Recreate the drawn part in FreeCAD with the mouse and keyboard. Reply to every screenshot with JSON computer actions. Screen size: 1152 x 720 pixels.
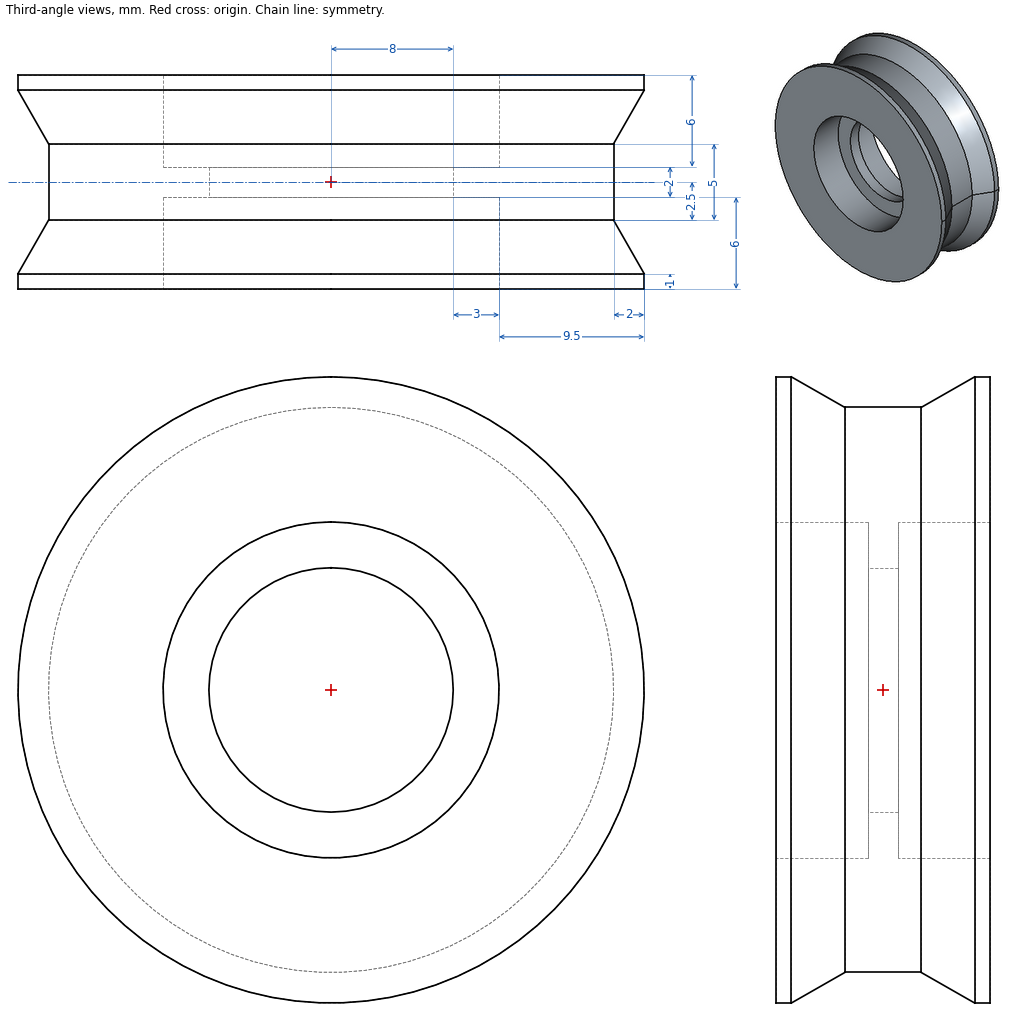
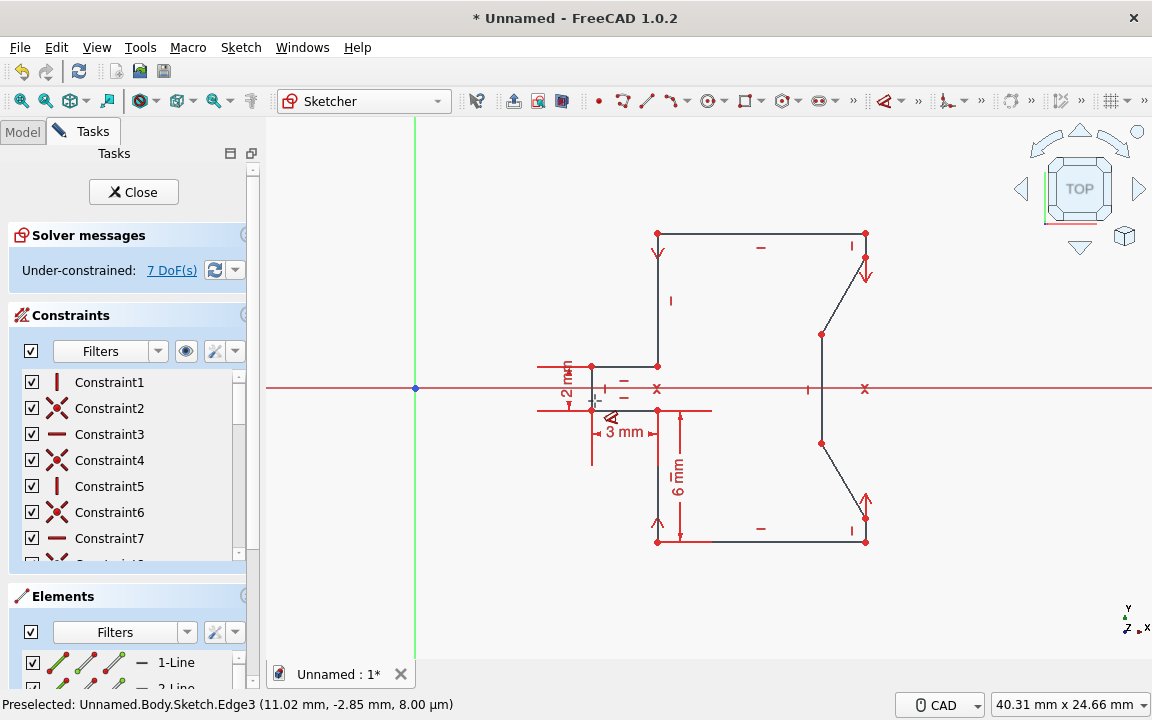
{"action": "scroll", "coordinate": [866, 535], "scroll_direction": "up", "scroll_amount": 4}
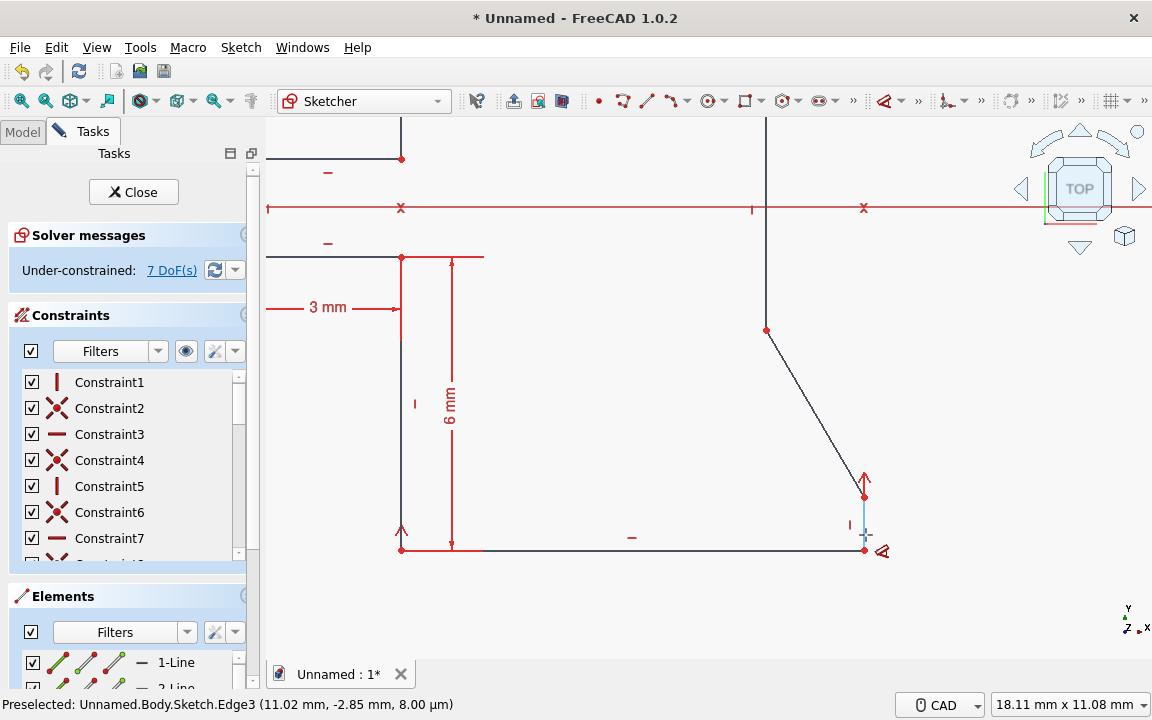
{"action": "left_click", "coordinate": [864, 535]}
{"action": "left_click", "coordinate": [898, 524]}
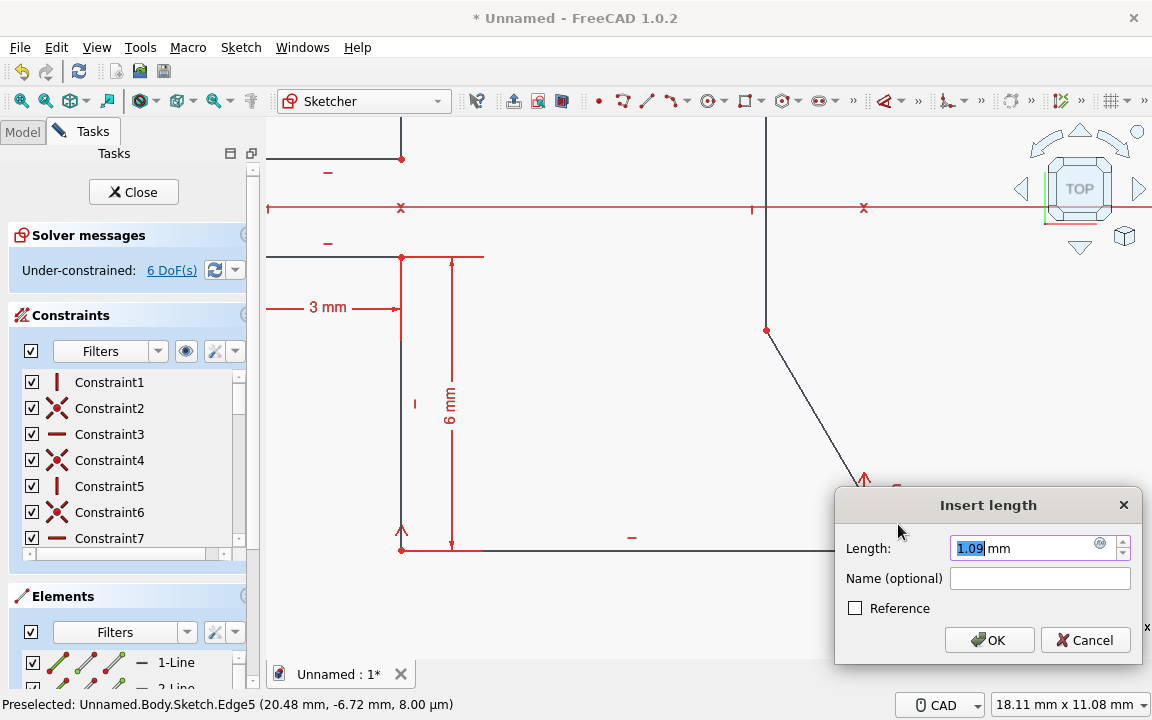
{"action": "type", "text": "1"}
{"action": "key", "text": "Return"}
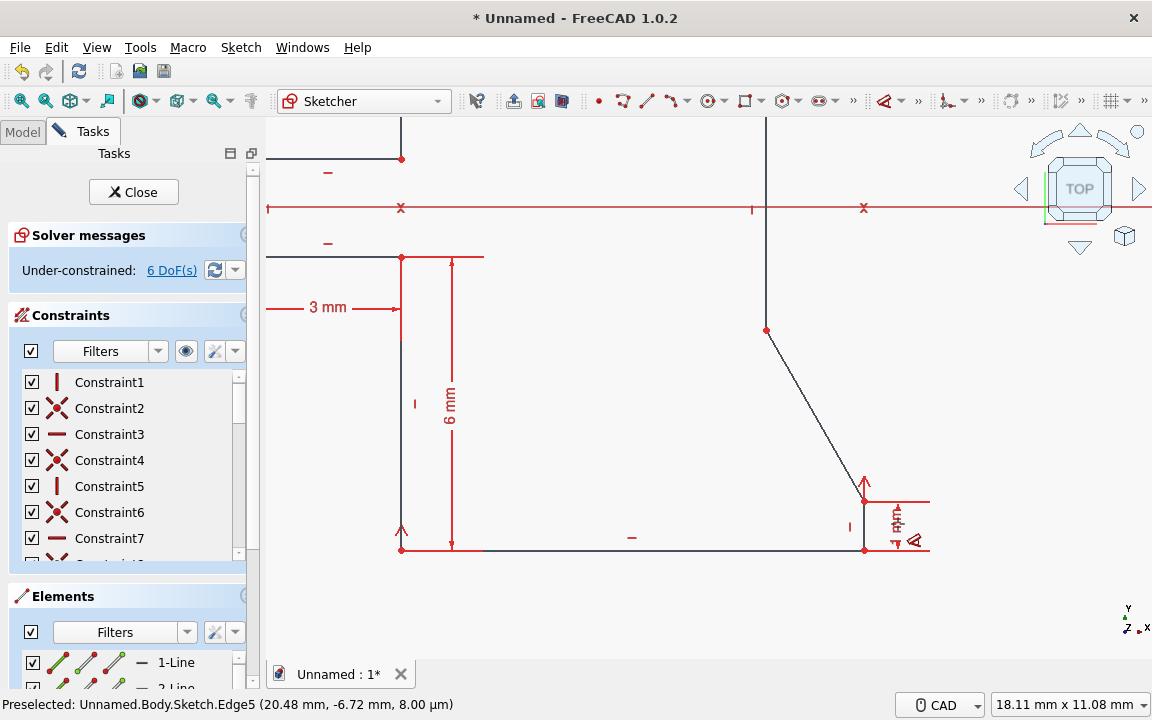
{"action": "left_click", "coordinate": [766, 258]}
{"action": "left_click", "coordinate": [800, 238]}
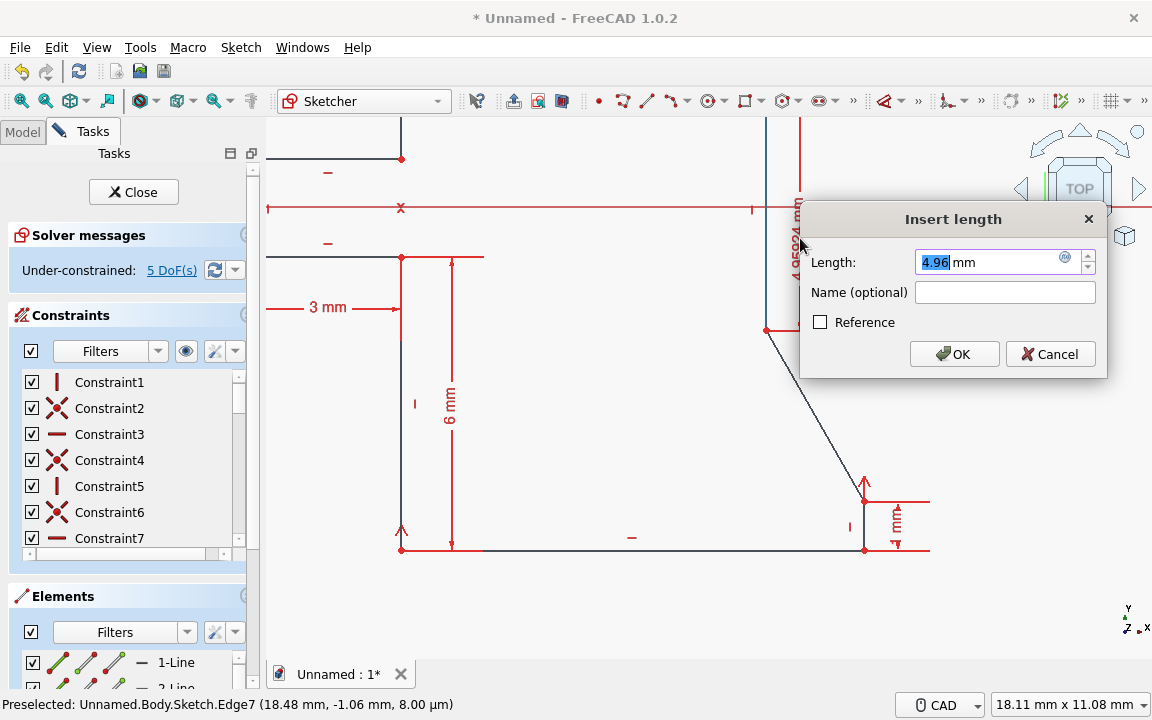
{"action": "type", "text": "5"}
{"action": "key", "text": "Return"}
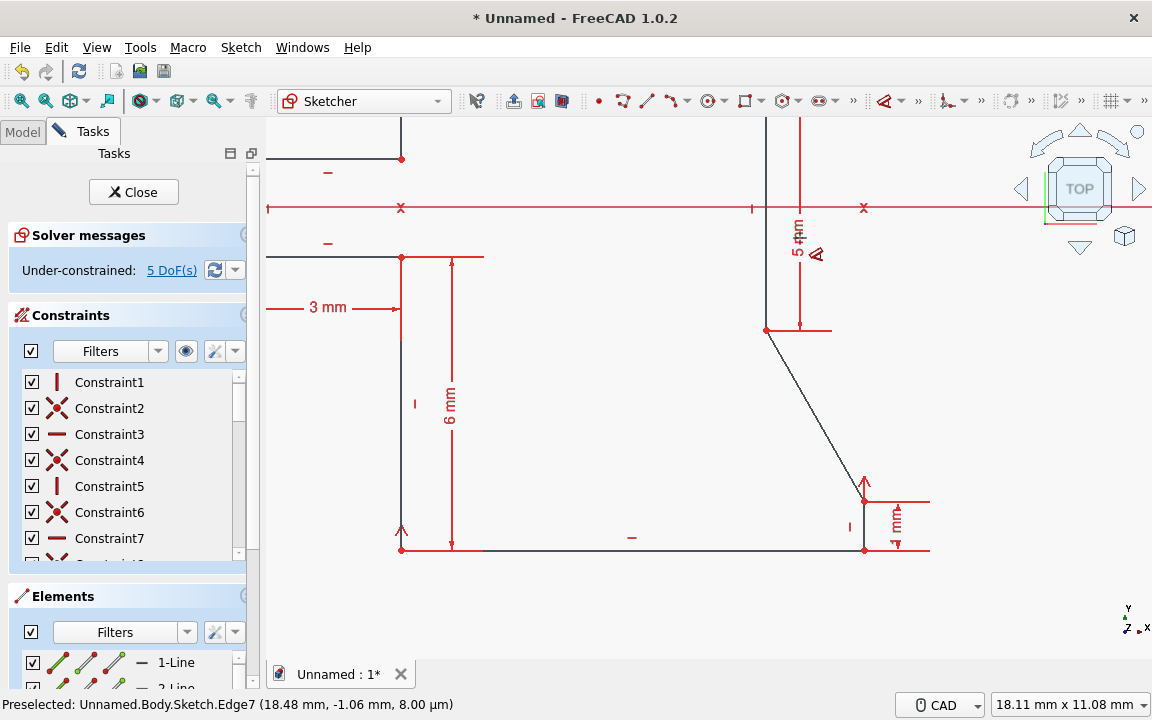
{"action": "scroll", "coordinate": [866, 536], "scroll_direction": "down", "scroll_amount": 4}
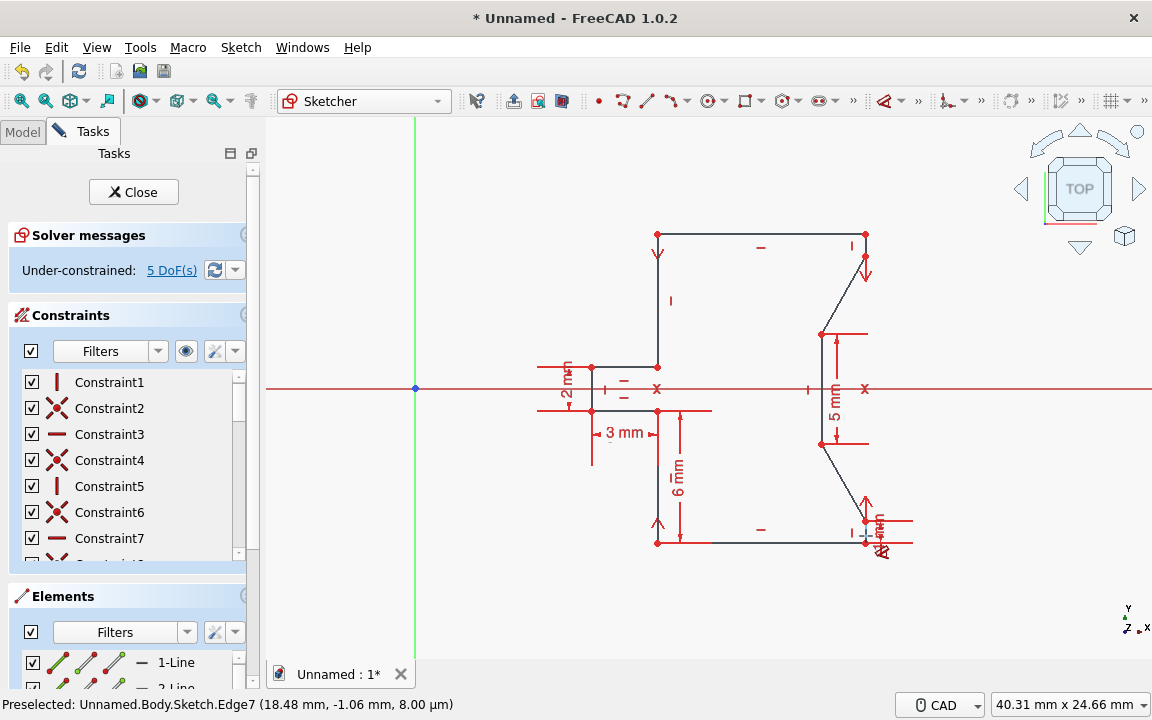
{"action": "left_click", "coordinate": [658, 274]}
{"action": "left_click", "coordinate": [692, 301]}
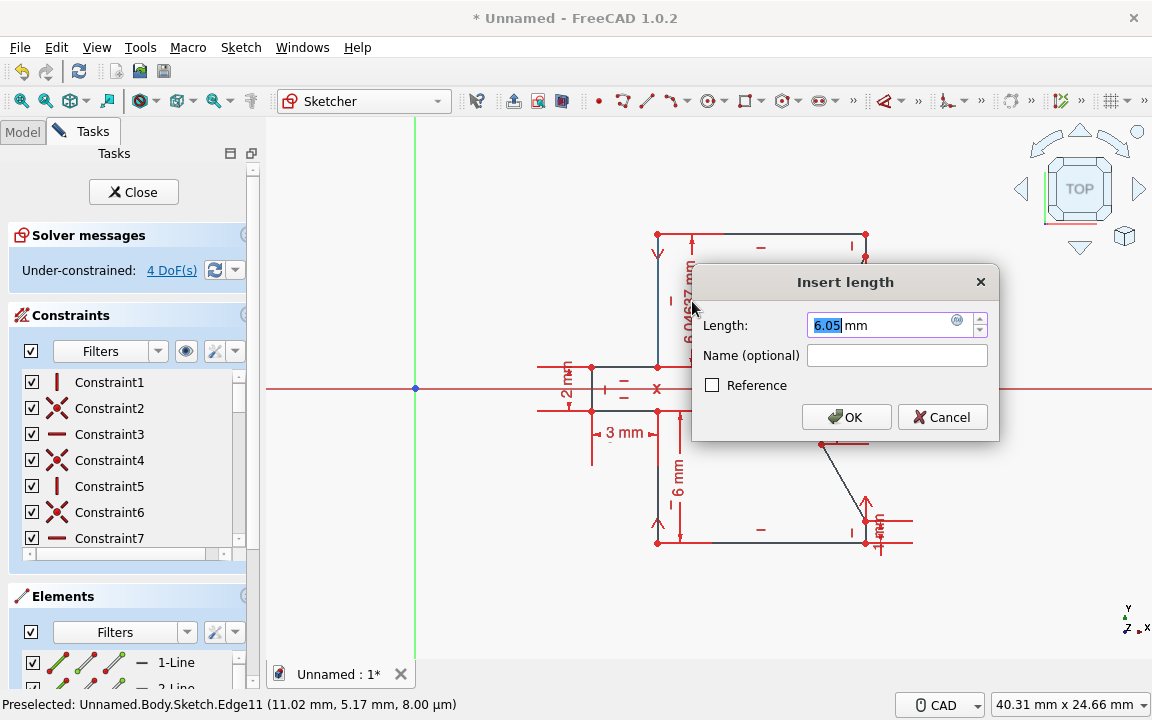
{"action": "type", "text": "6"}
{"action": "key", "text": "Return"}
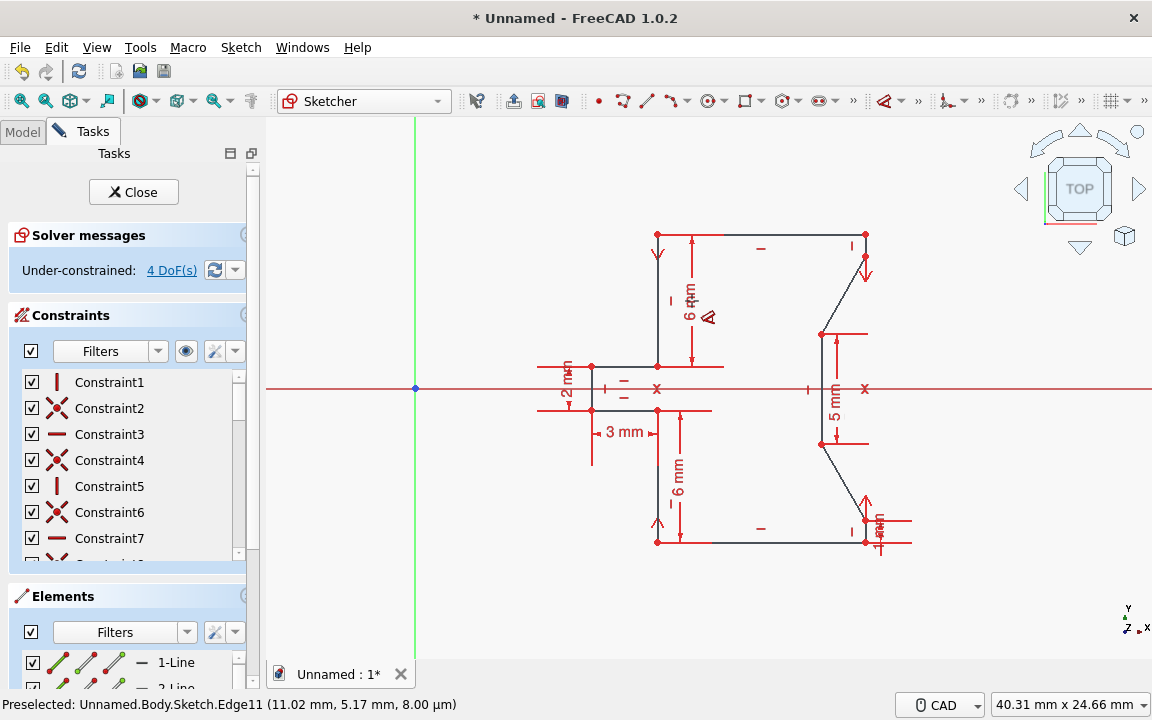
{"action": "left_click", "coordinate": [592, 367]}
{"action": "left_click", "coordinate": [504, 333]}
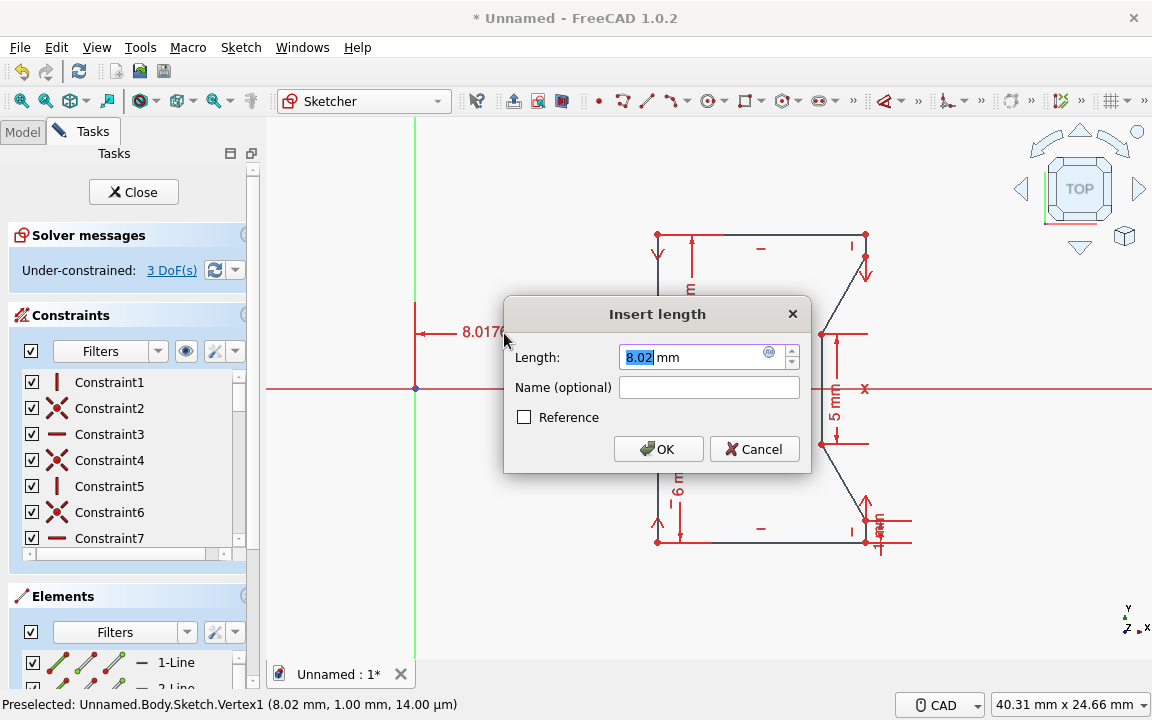
{"action": "type", "text": "8"}
{"action": "key", "text": "Return"}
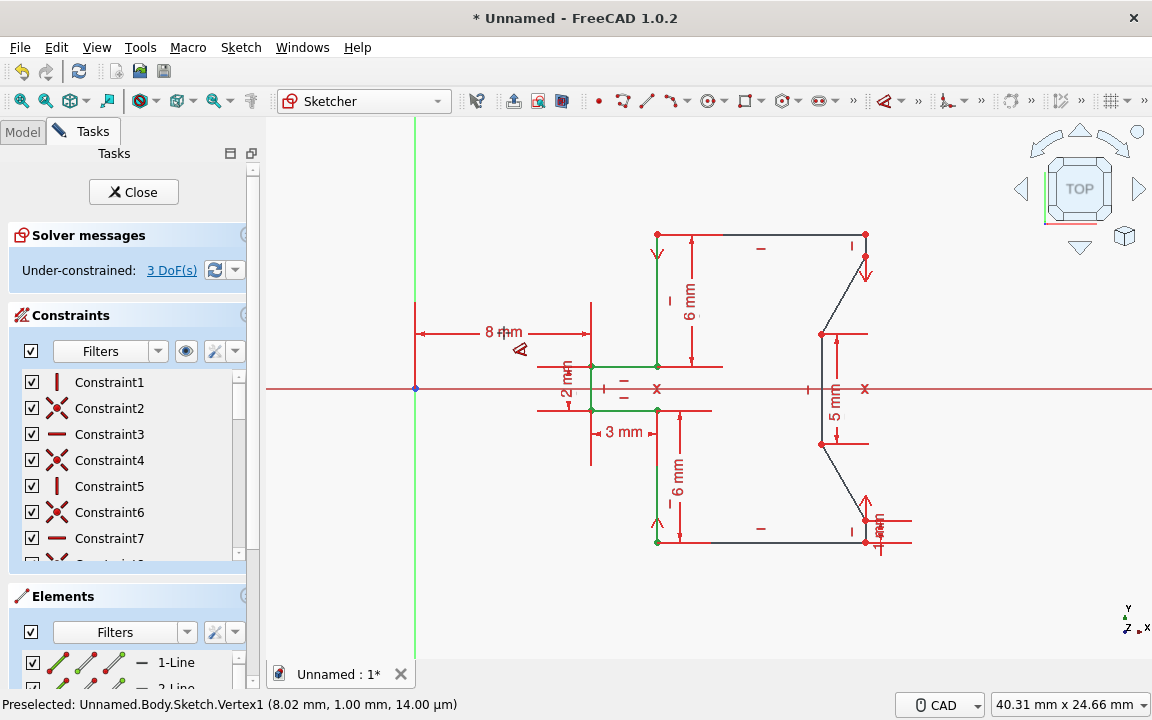
{"action": "left_click", "coordinate": [852, 498]}
{"action": "left_click", "coordinate": [844, 579]}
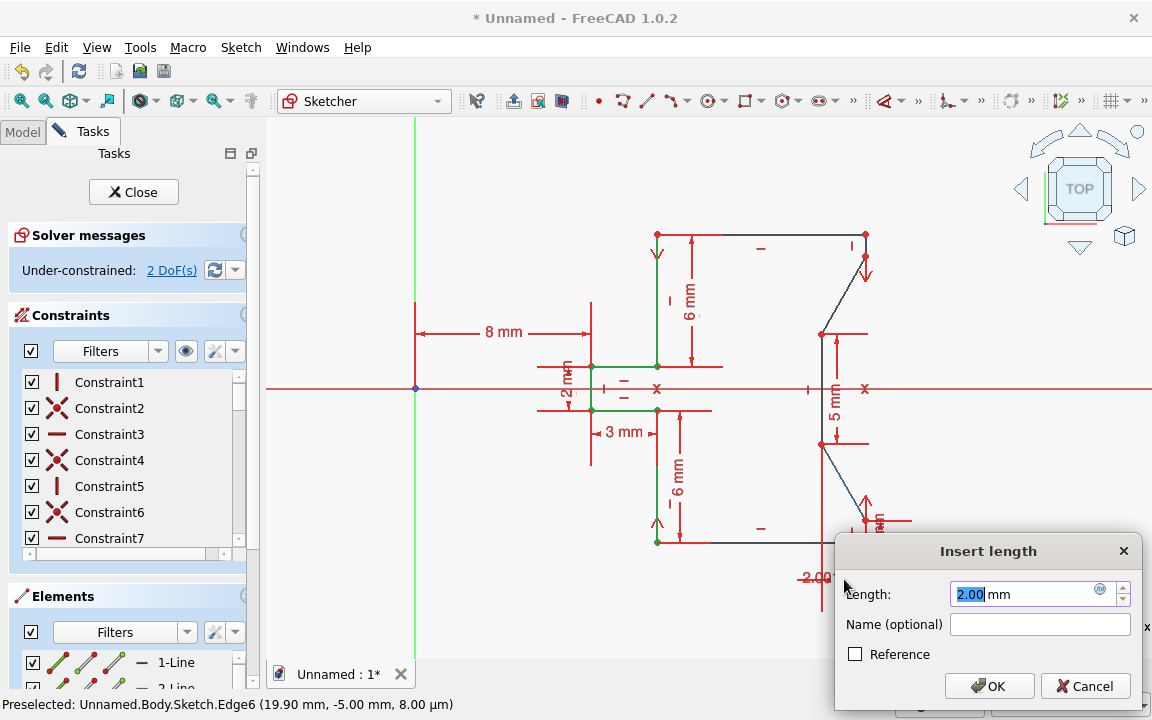
{"action": "type", "text": "2"}
{"action": "key", "text": "Return"}